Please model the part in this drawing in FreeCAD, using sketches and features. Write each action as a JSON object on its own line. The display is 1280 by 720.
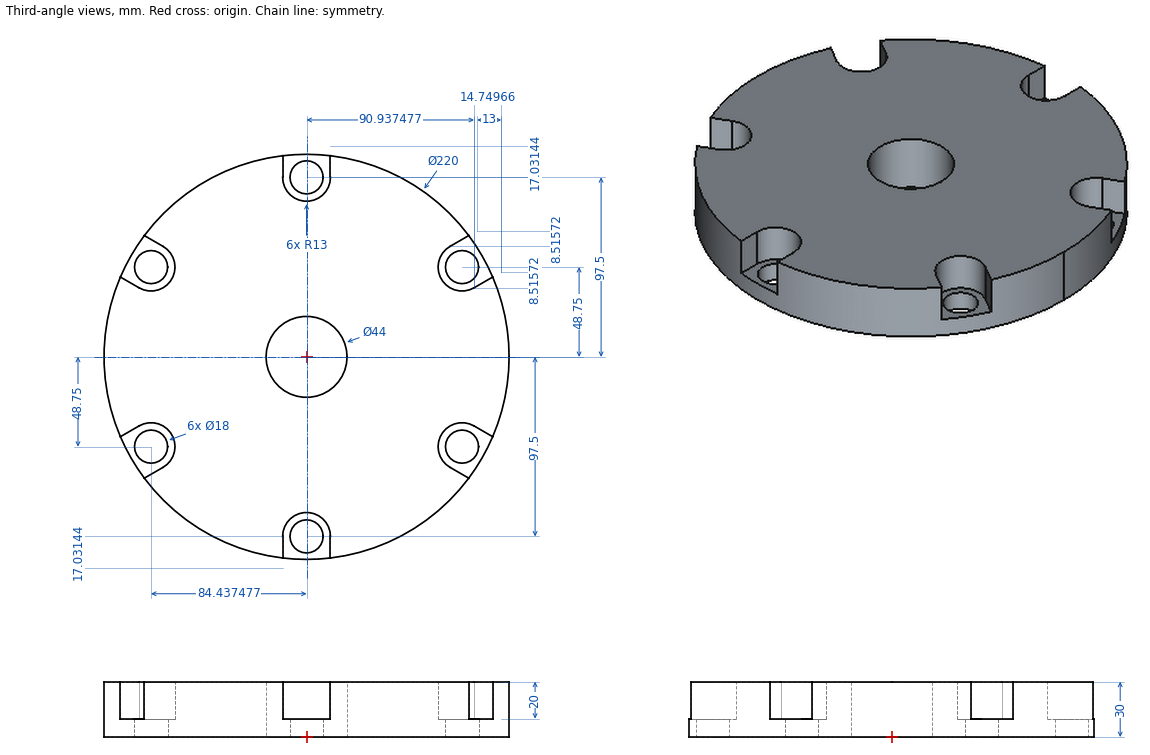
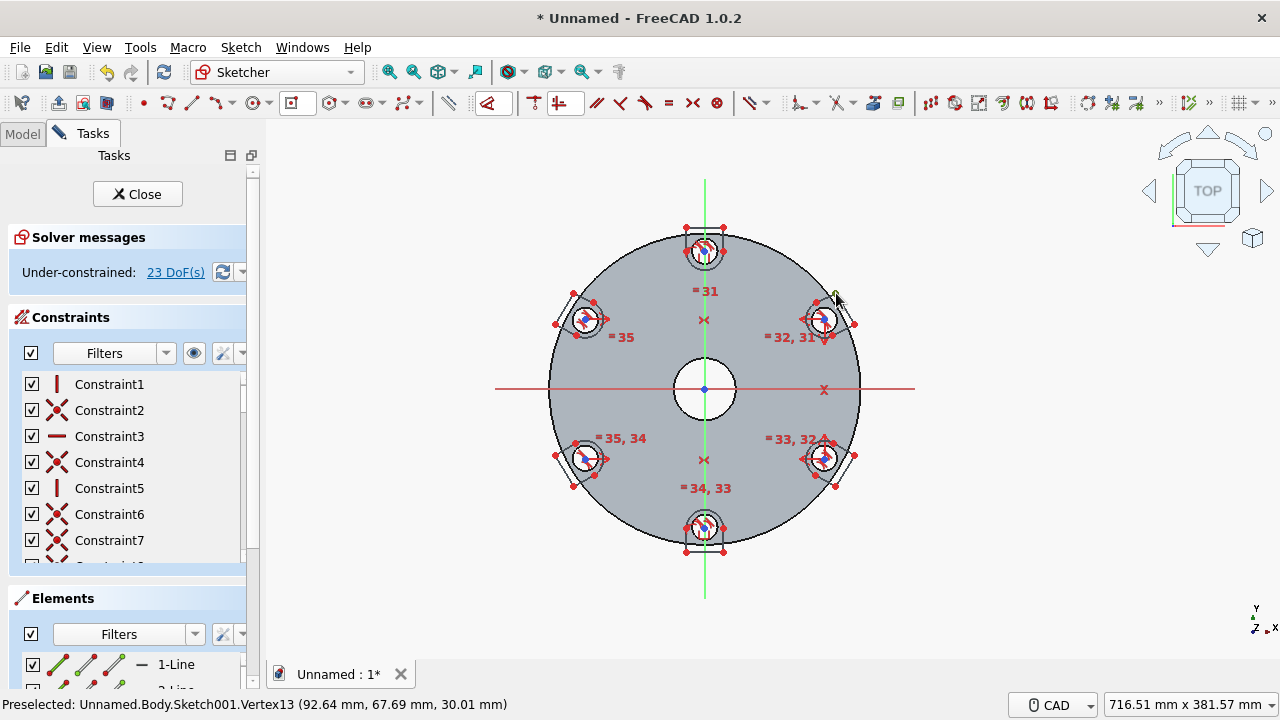
{"action": "left_click", "coordinate": [836, 487]}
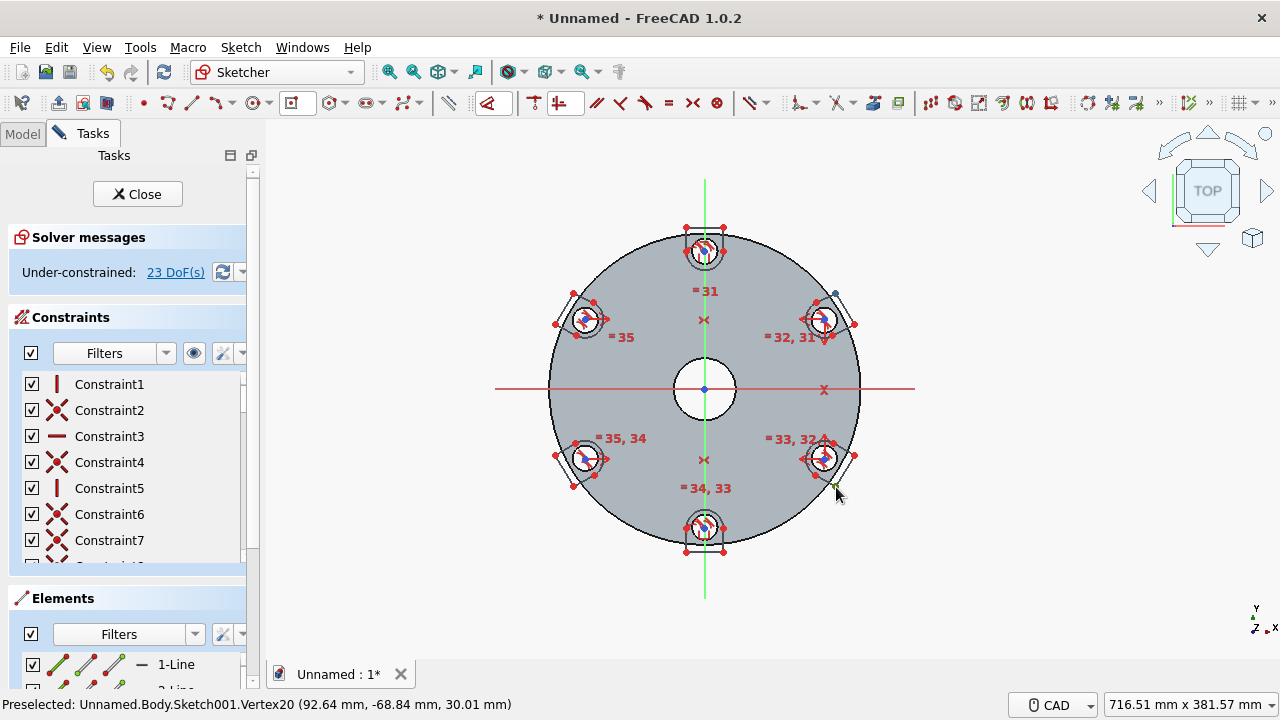
{"action": "left_click", "coordinate": [529, 389]}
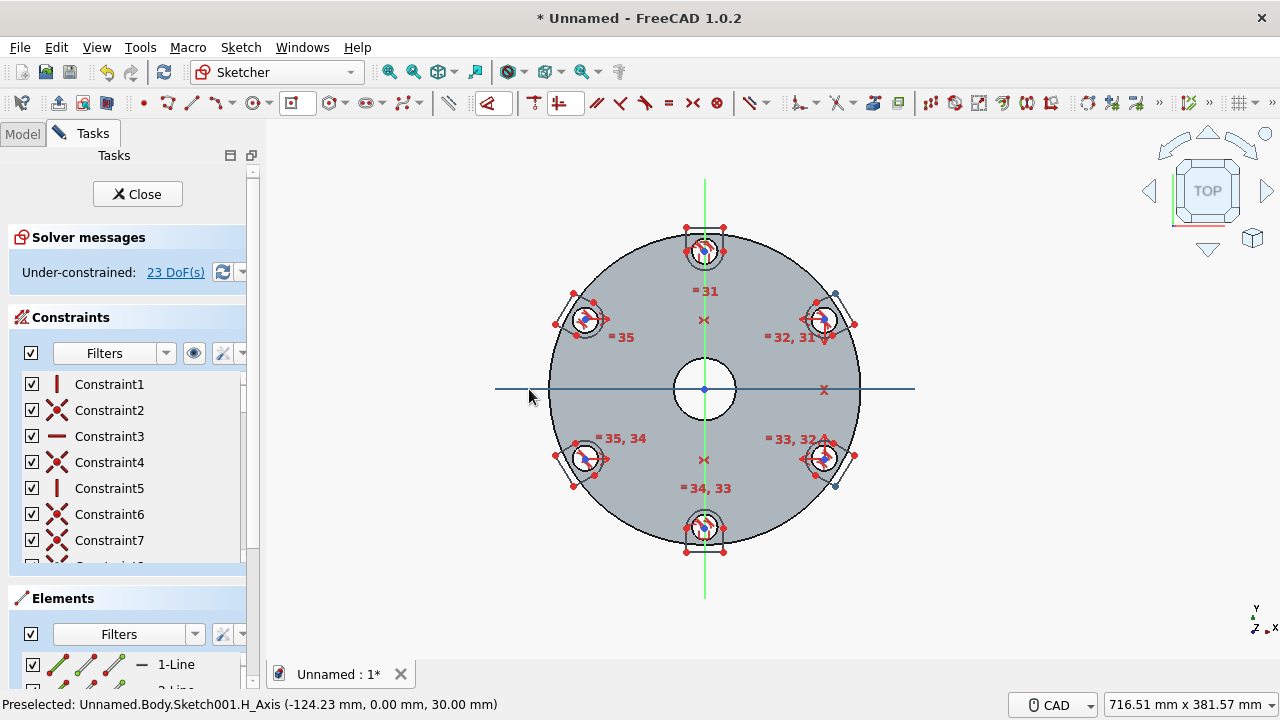
{"action": "key", "text": "s"}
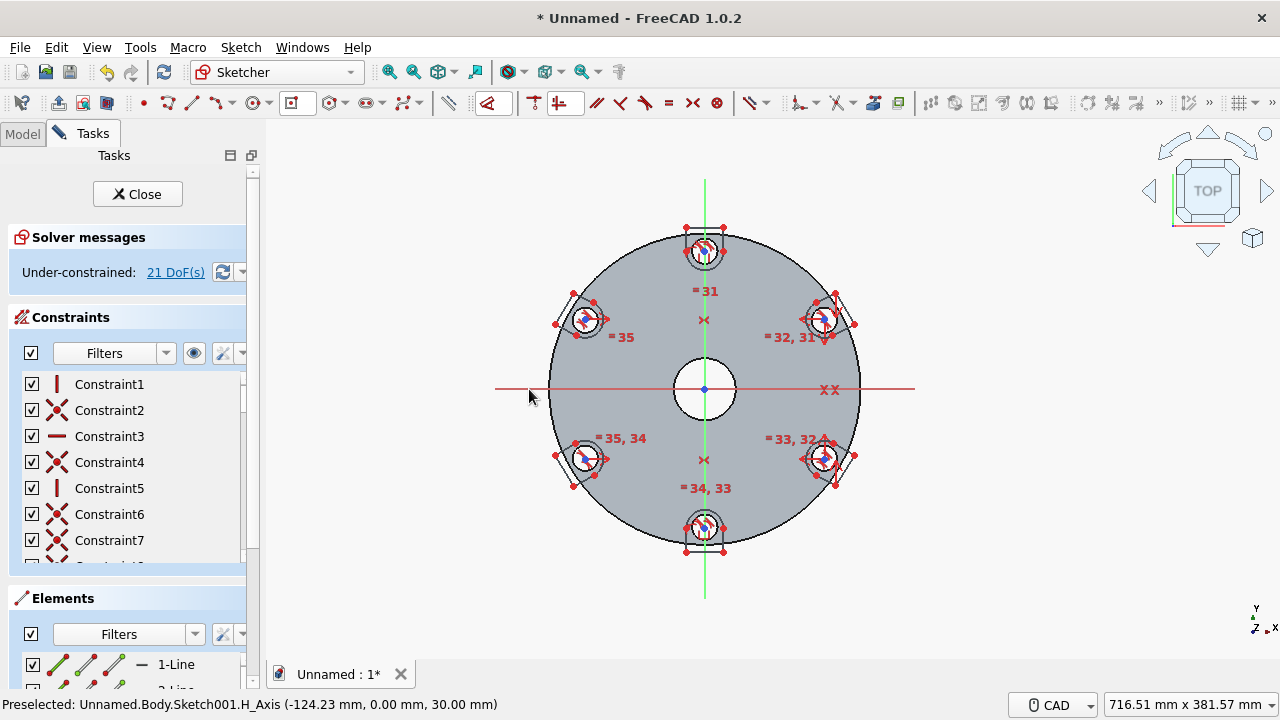
{"action": "left_click", "coordinate": [855, 325]}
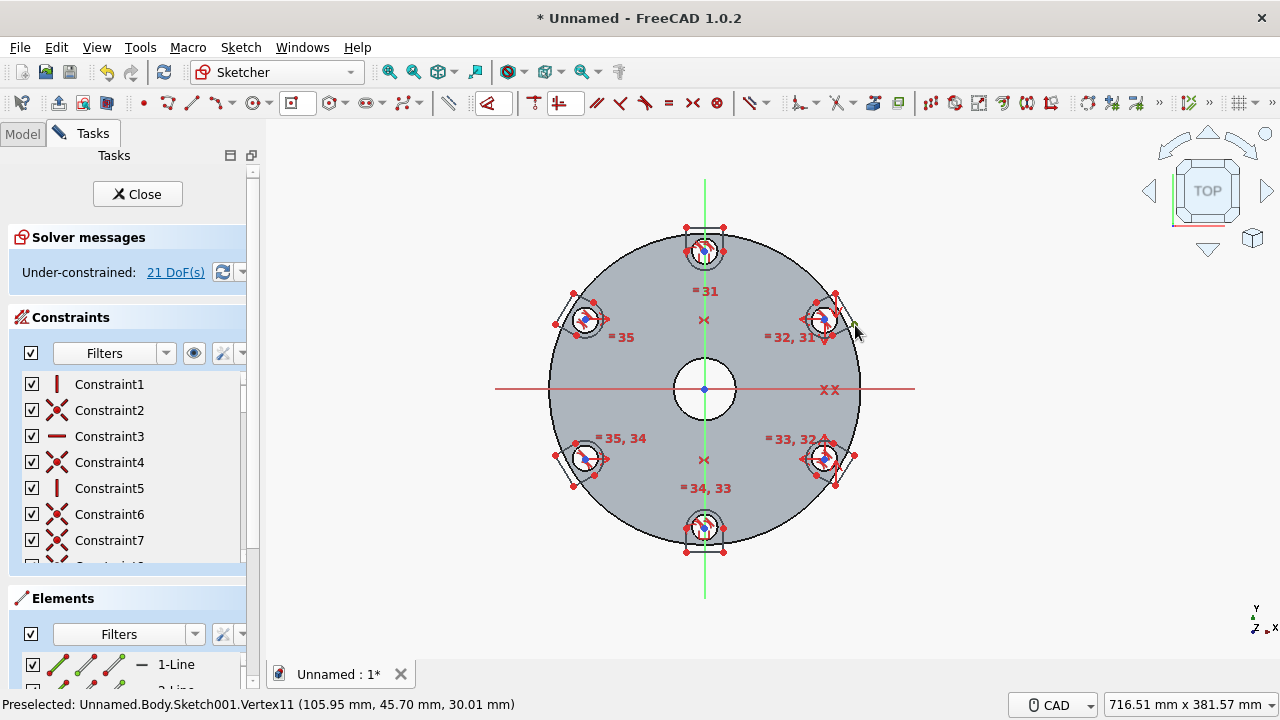
{"action": "left_click", "coordinate": [855, 456]}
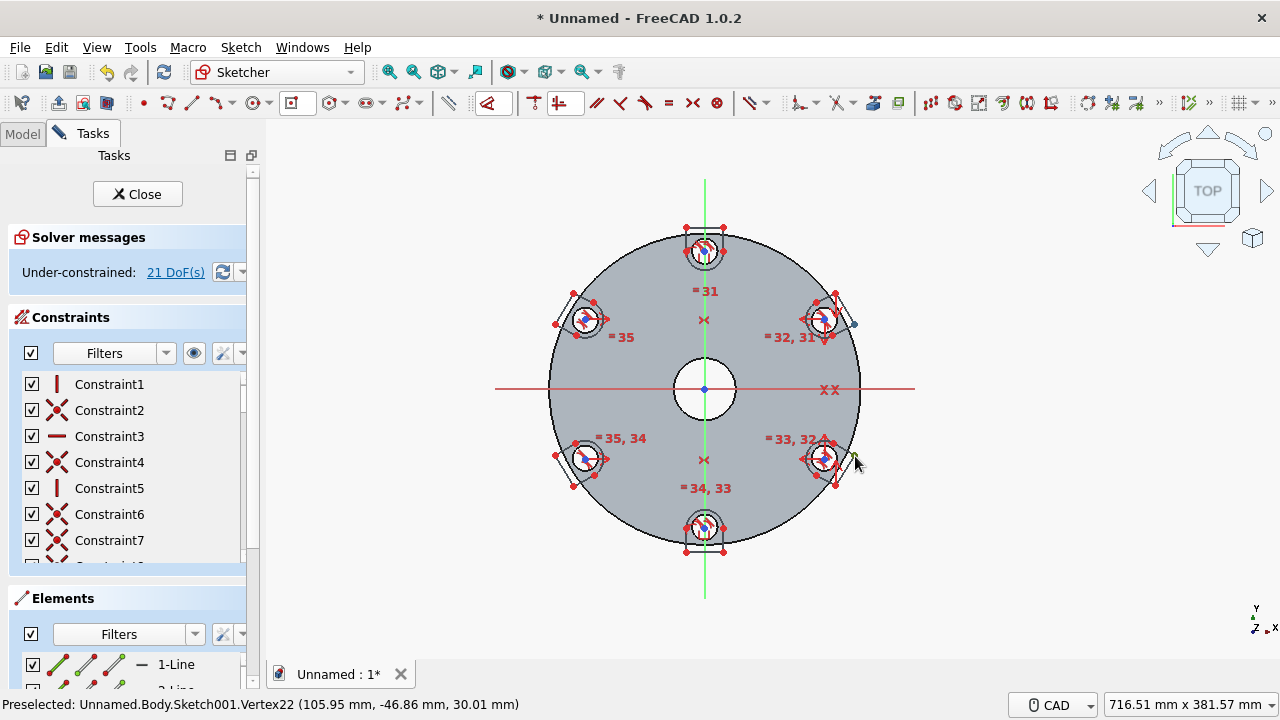
{"action": "left_click", "coordinate": [529, 389]}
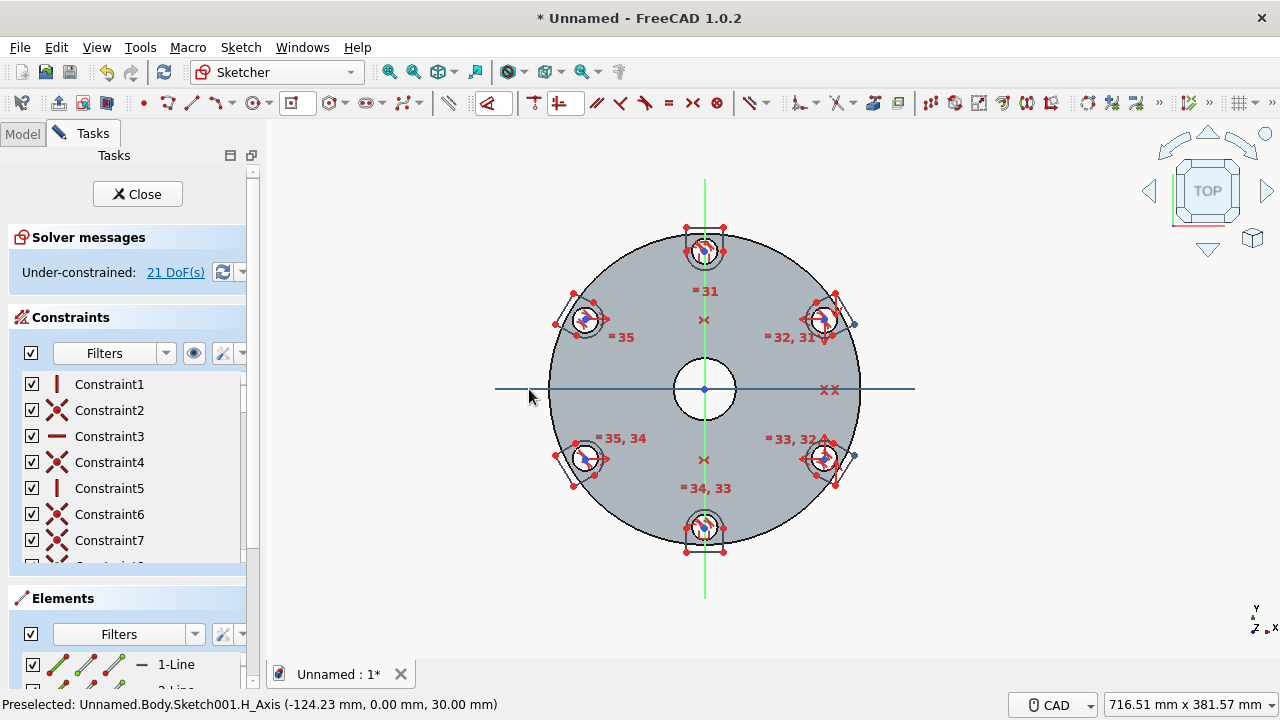
{"action": "left_click", "coordinate": [694, 104]}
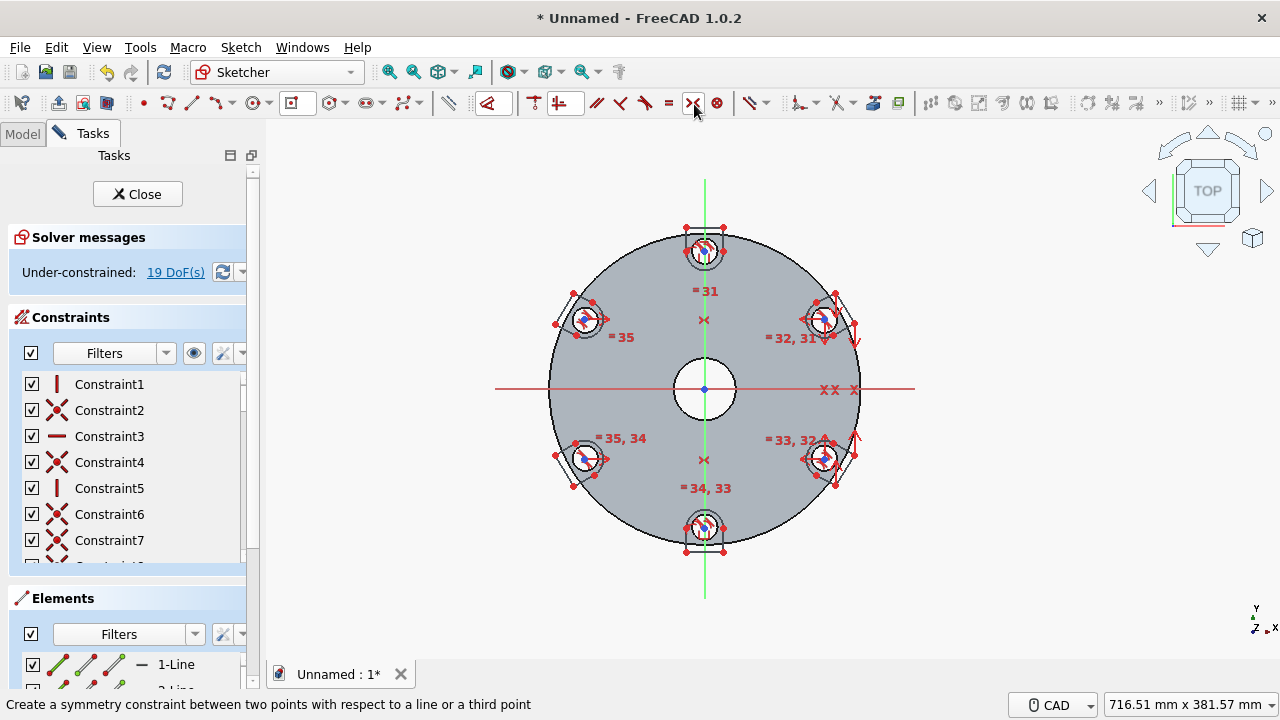
{"action": "left_click", "coordinate": [855, 455]}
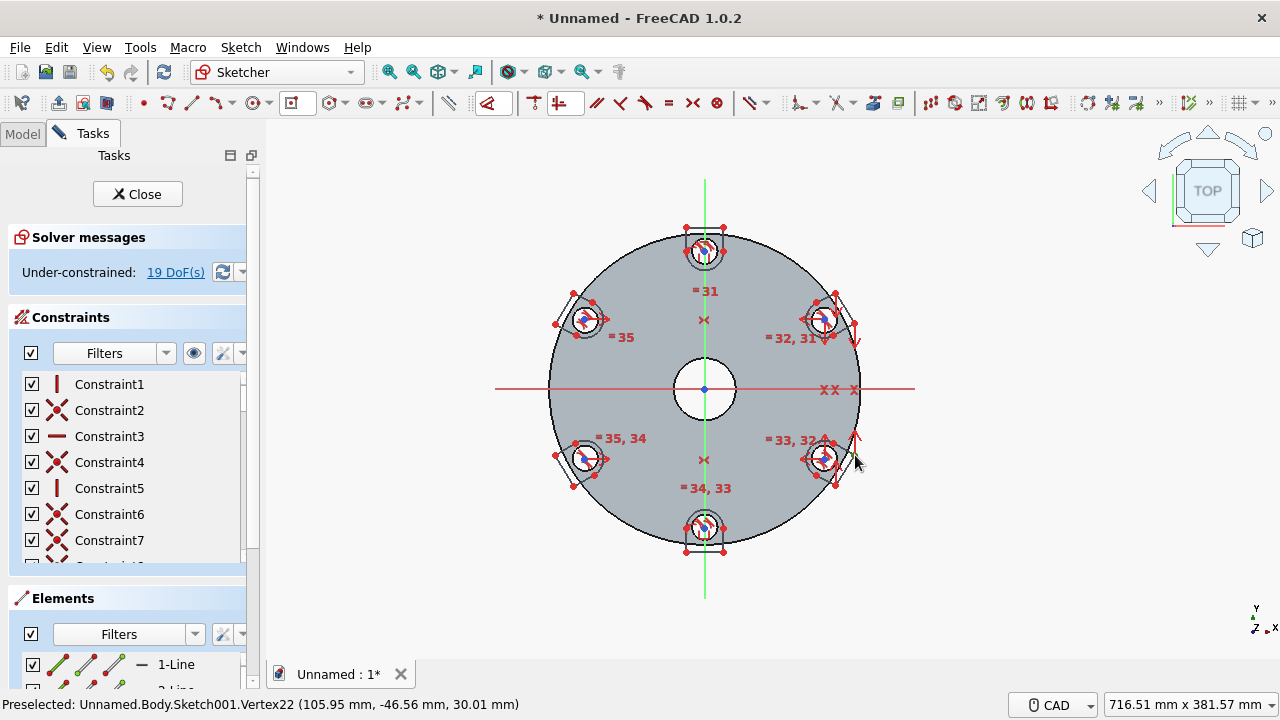
{"action": "left_click", "coordinate": [555, 456]}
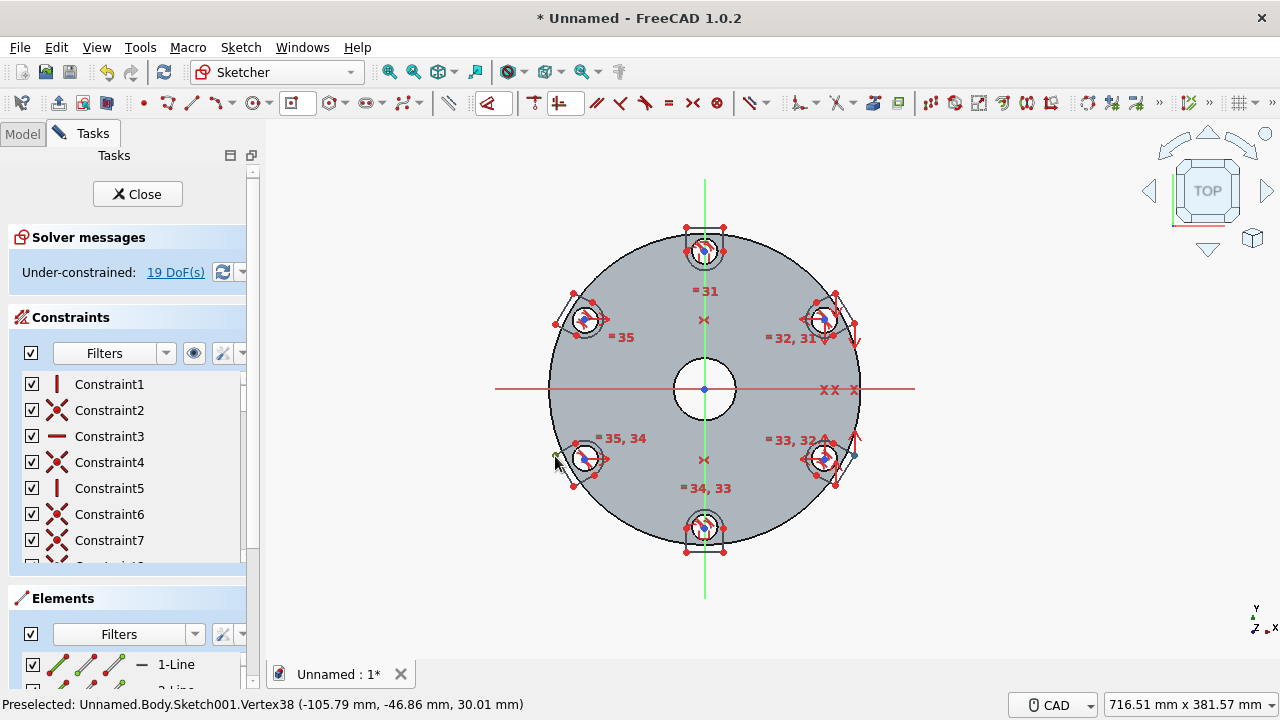
{"action": "left_click", "coordinate": [705, 596]}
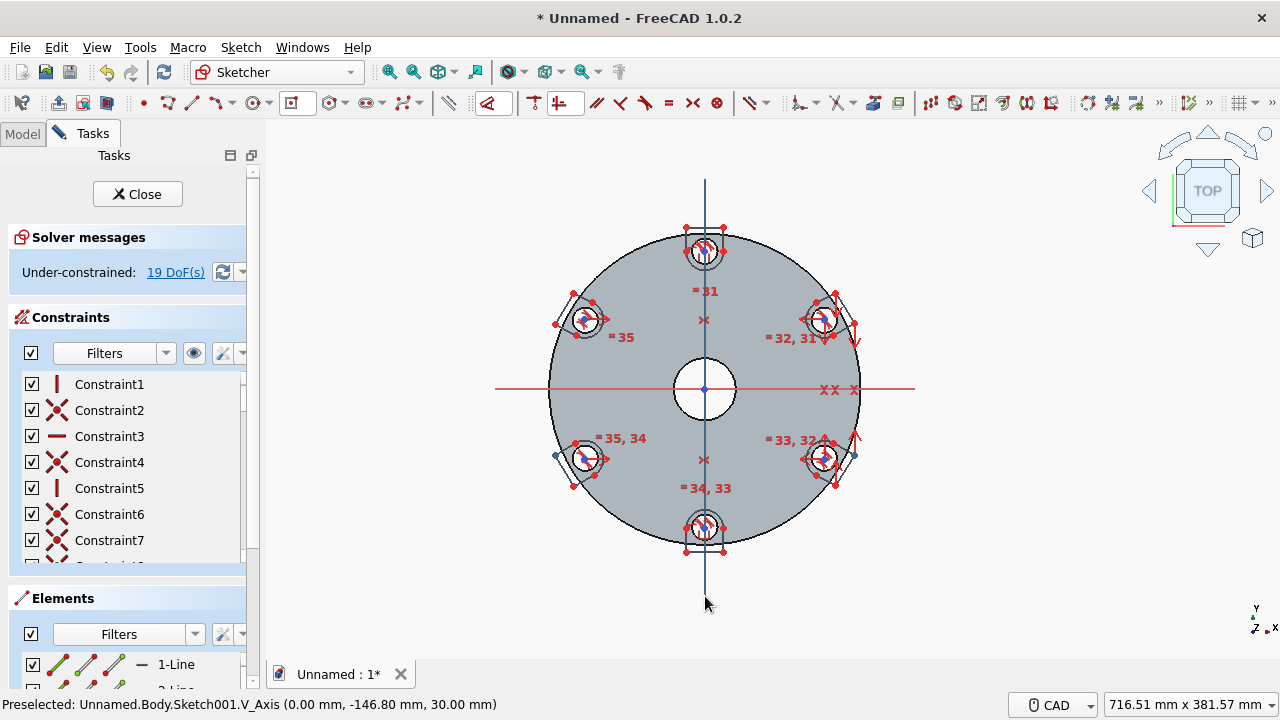
{"action": "left_click", "coordinate": [694, 104]}